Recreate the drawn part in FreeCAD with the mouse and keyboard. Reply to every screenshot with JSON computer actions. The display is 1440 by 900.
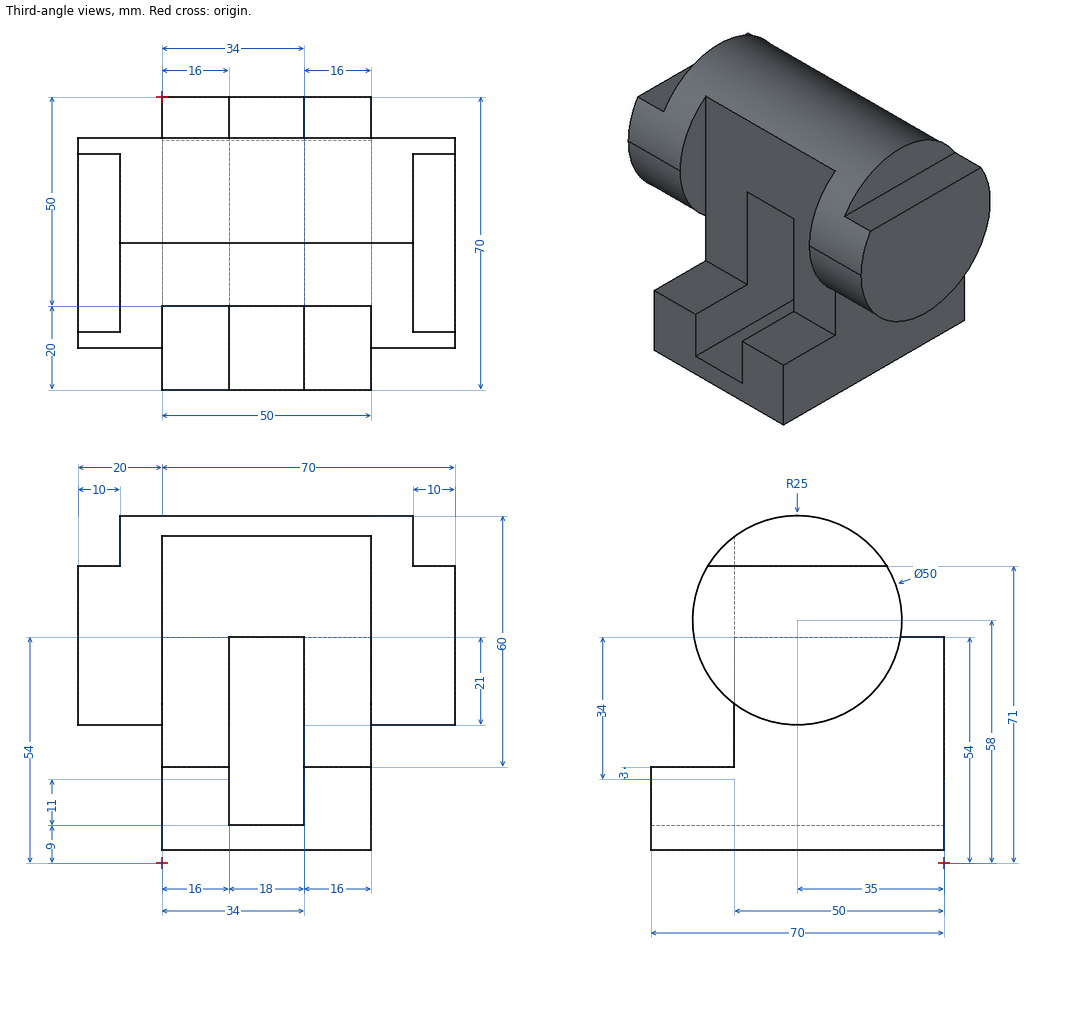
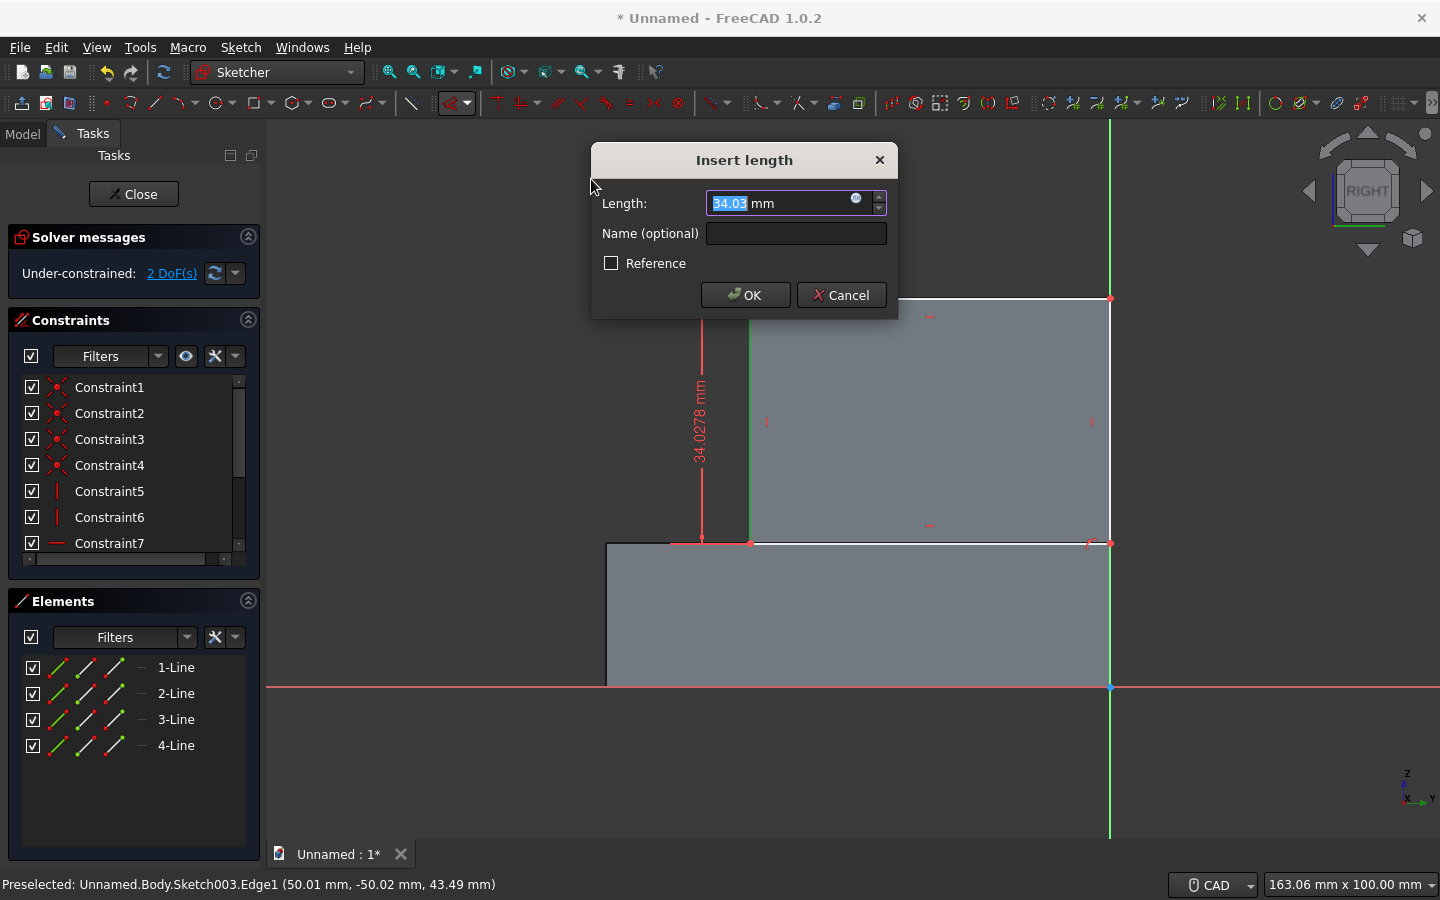
{"action": "type", "text": "34"}
{"action": "key", "text": "Return"}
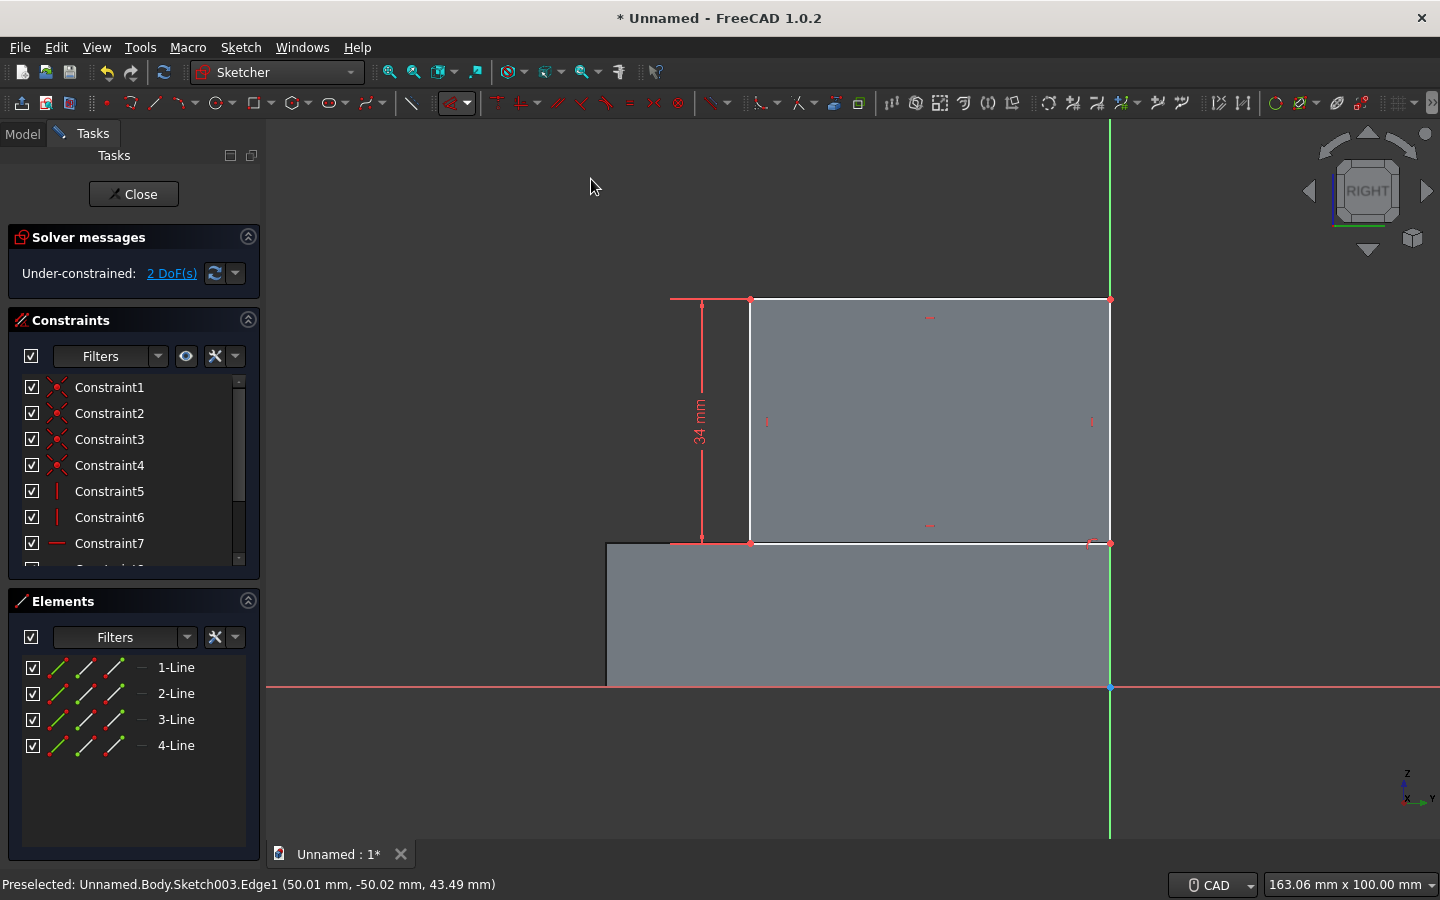
{"action": "left_click", "coordinate": [858, 544]}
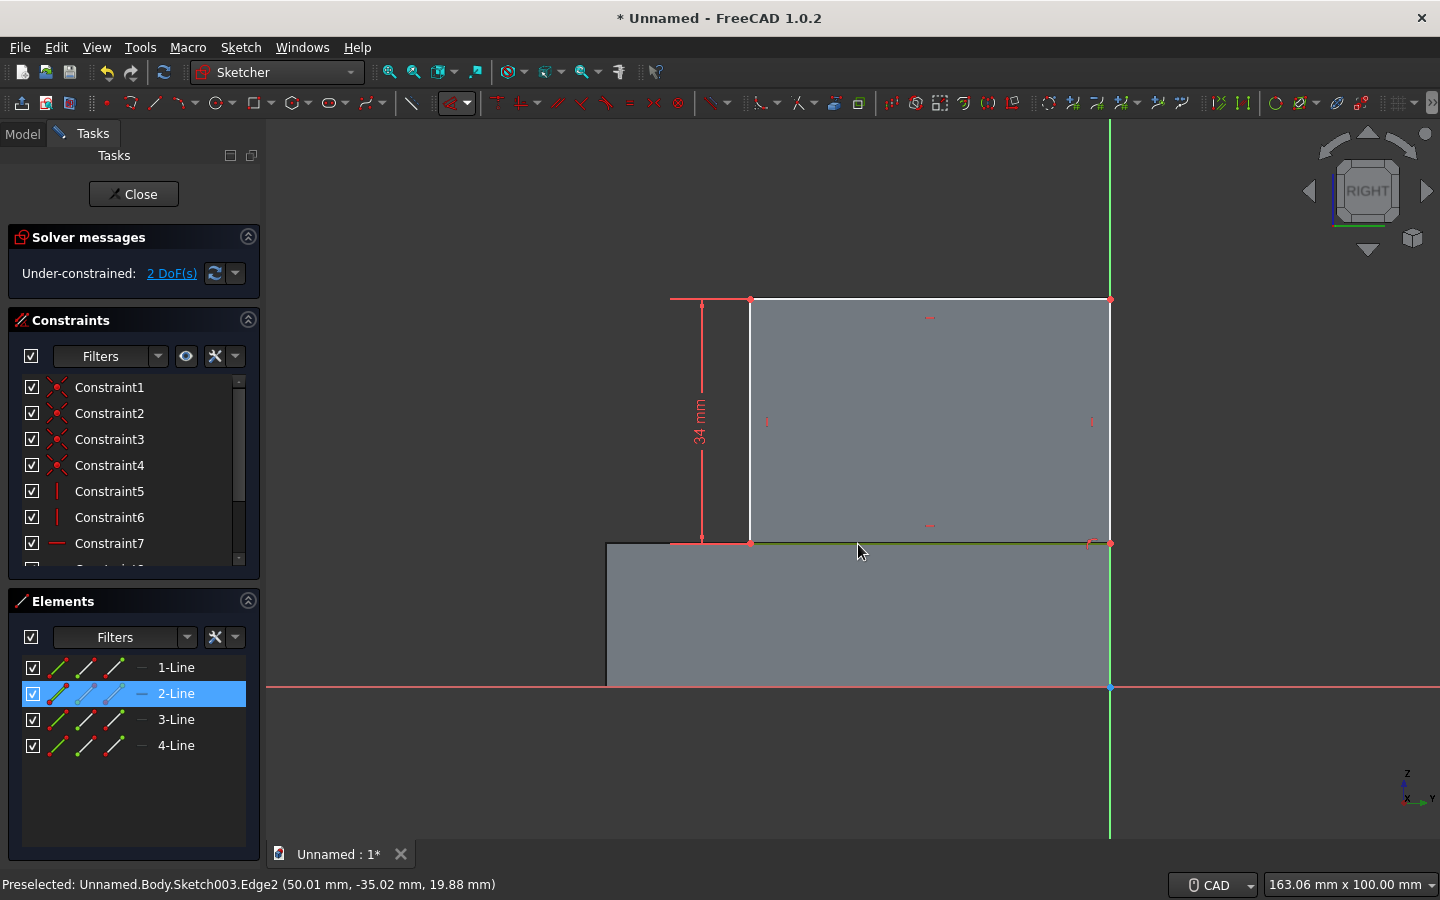
{"action": "key", "text": "l"}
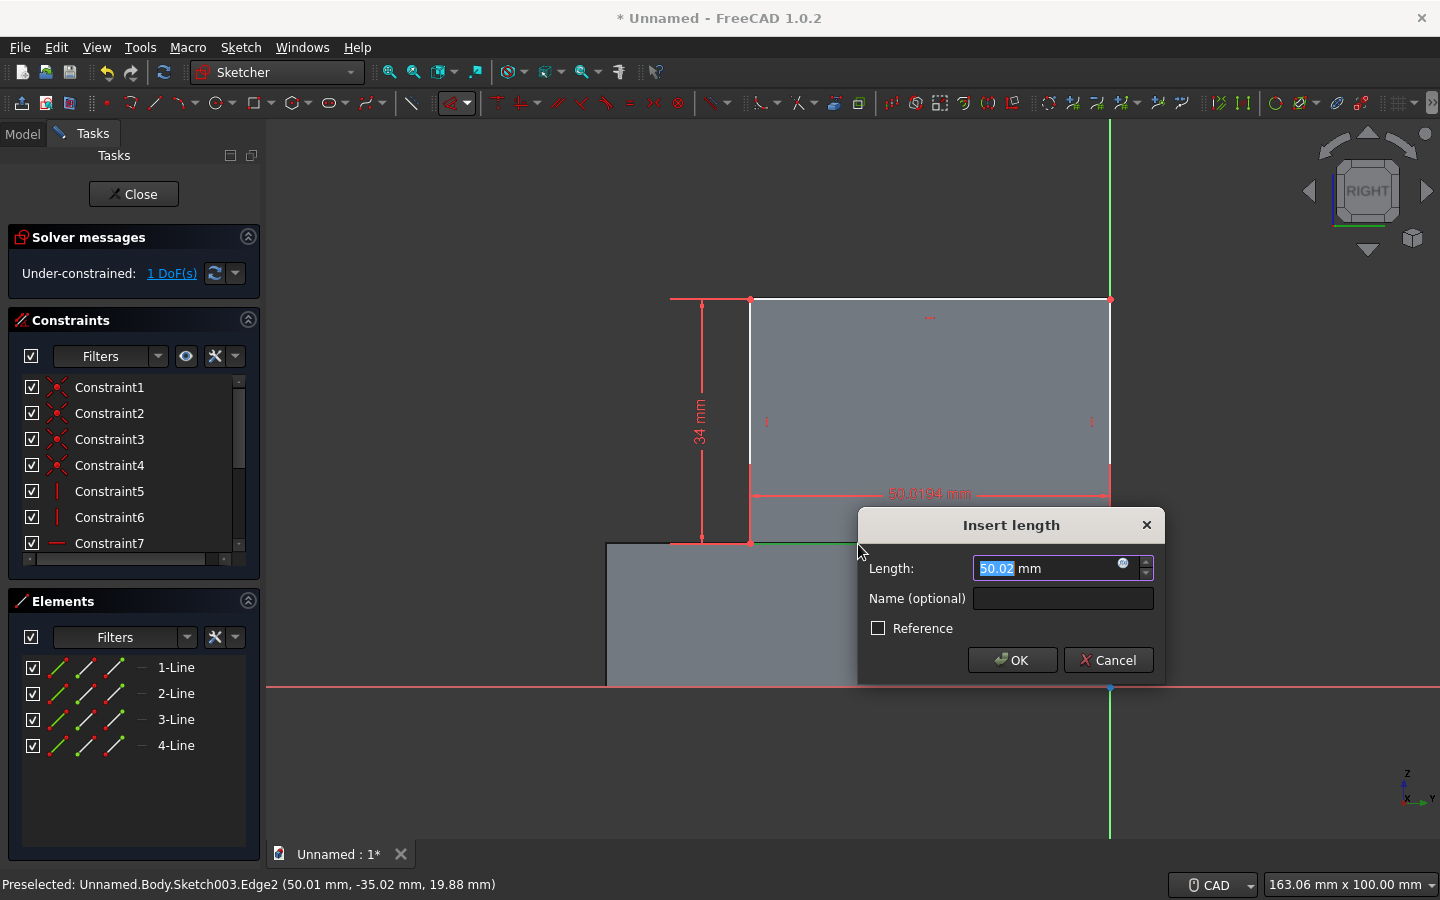
{"action": "type", "text": "50"}
{"action": "key", "text": "Return"}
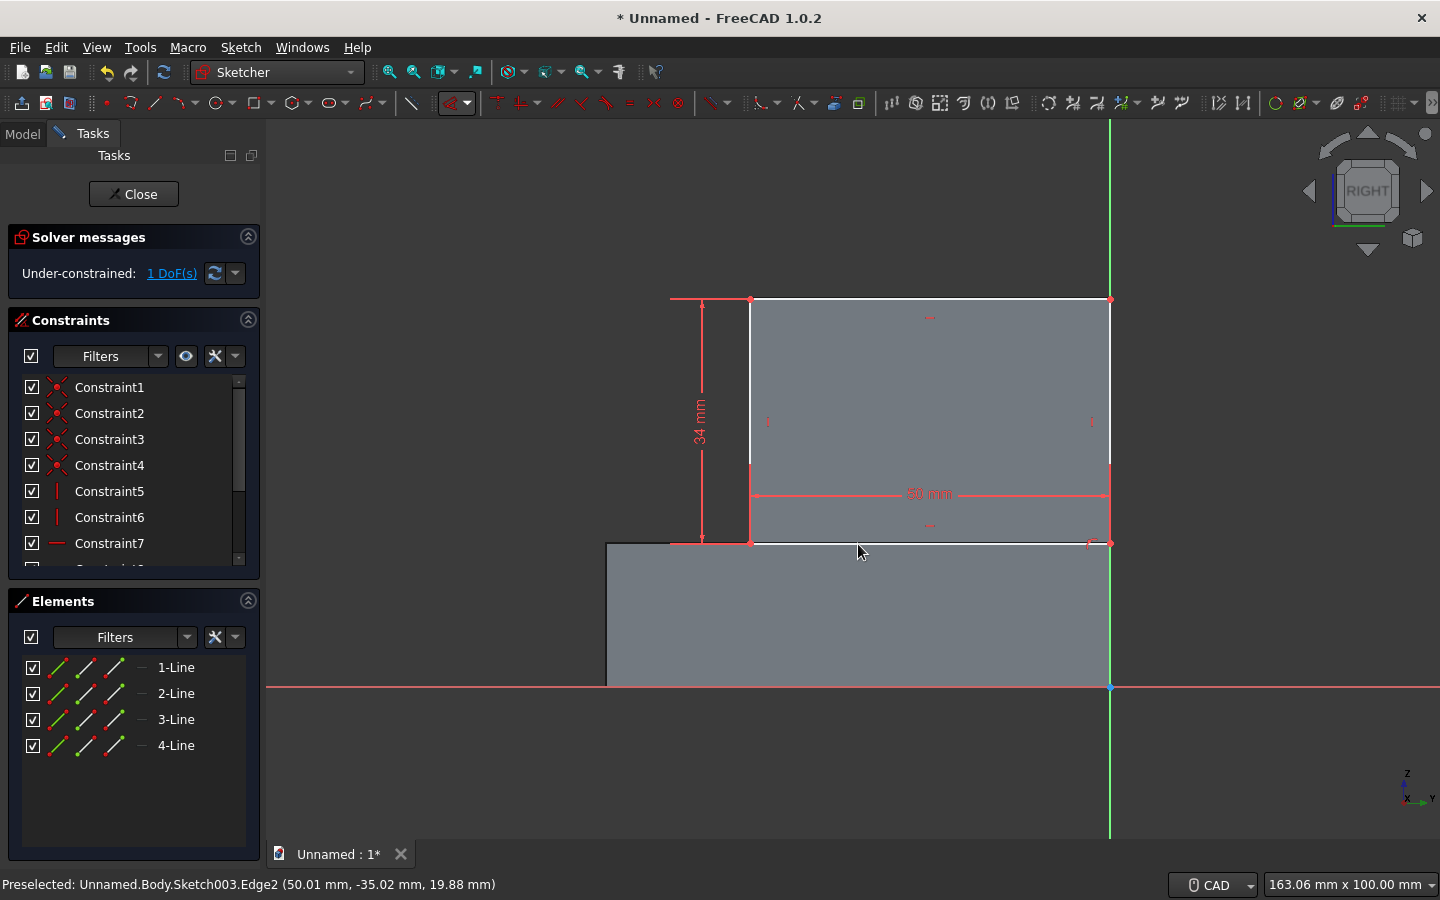
{"action": "left_click", "coordinate": [750, 299]}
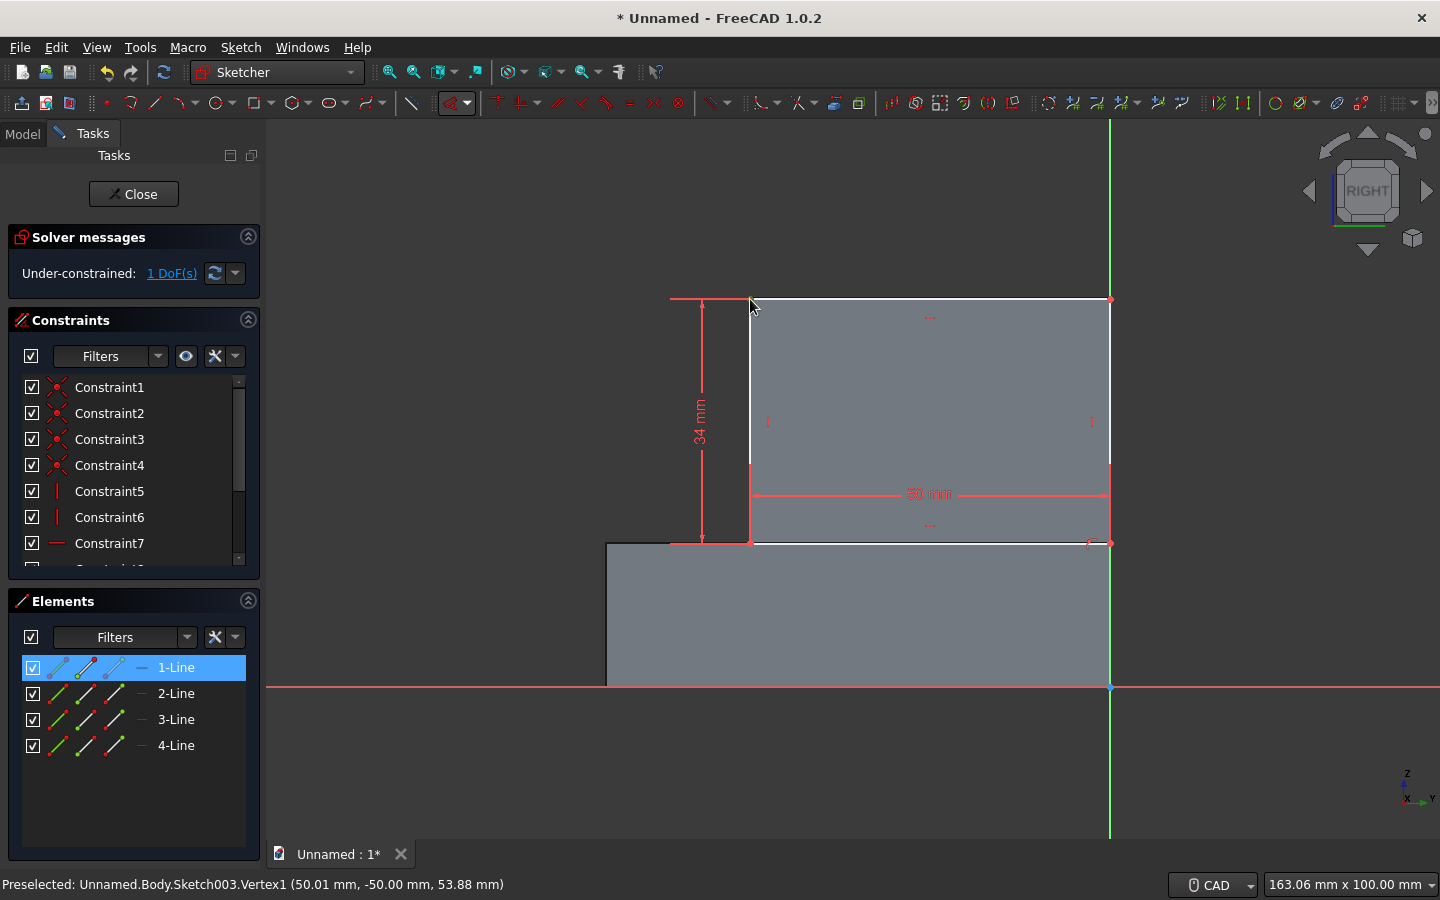
{"action": "key", "text": "i"}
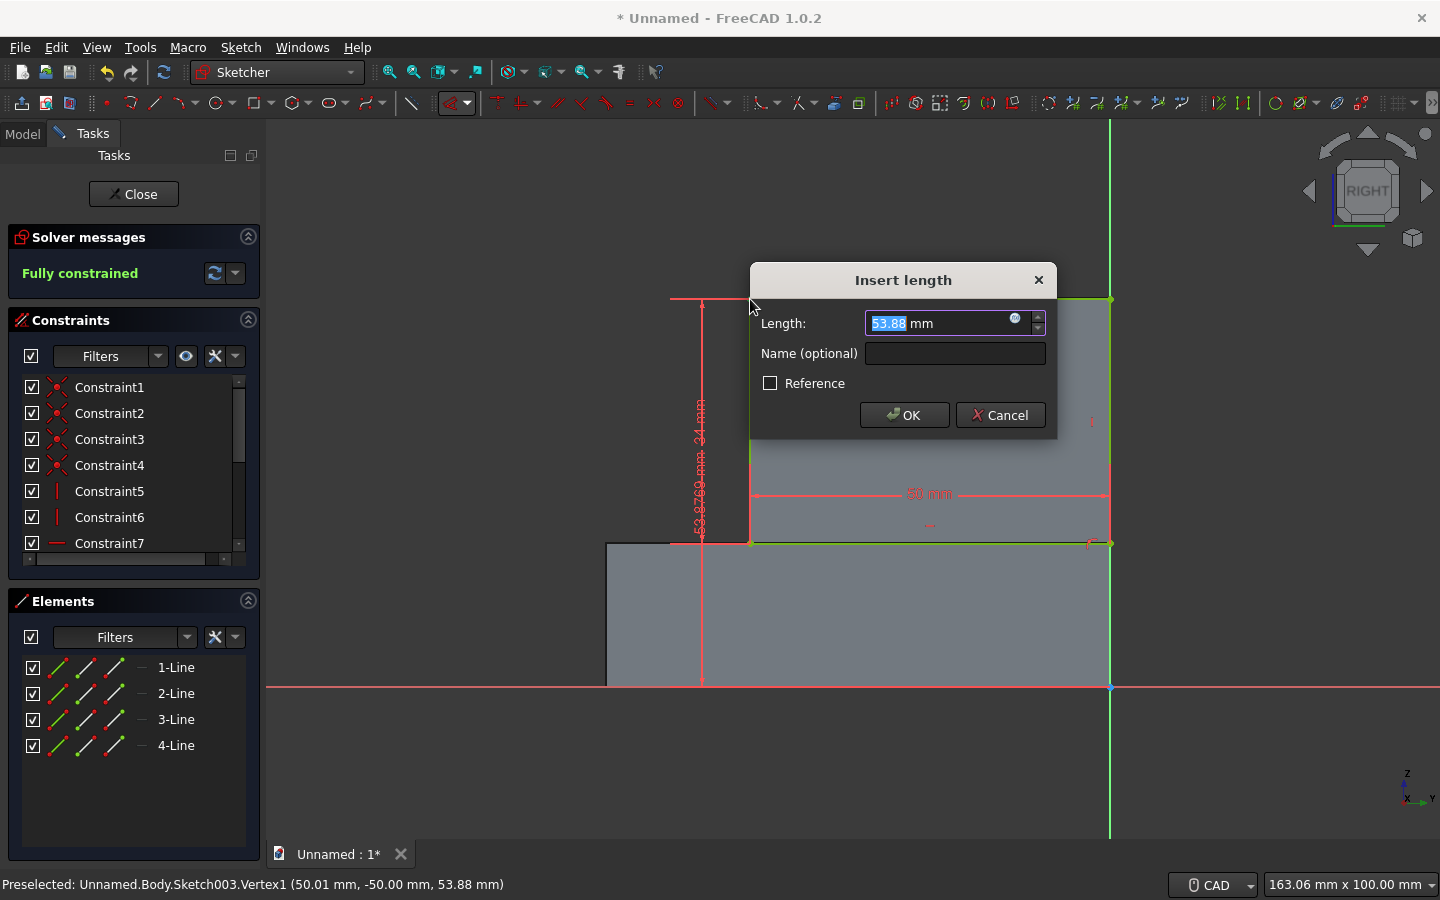
{"action": "type", "text": "54"}
{"action": "key", "text": "Return"}